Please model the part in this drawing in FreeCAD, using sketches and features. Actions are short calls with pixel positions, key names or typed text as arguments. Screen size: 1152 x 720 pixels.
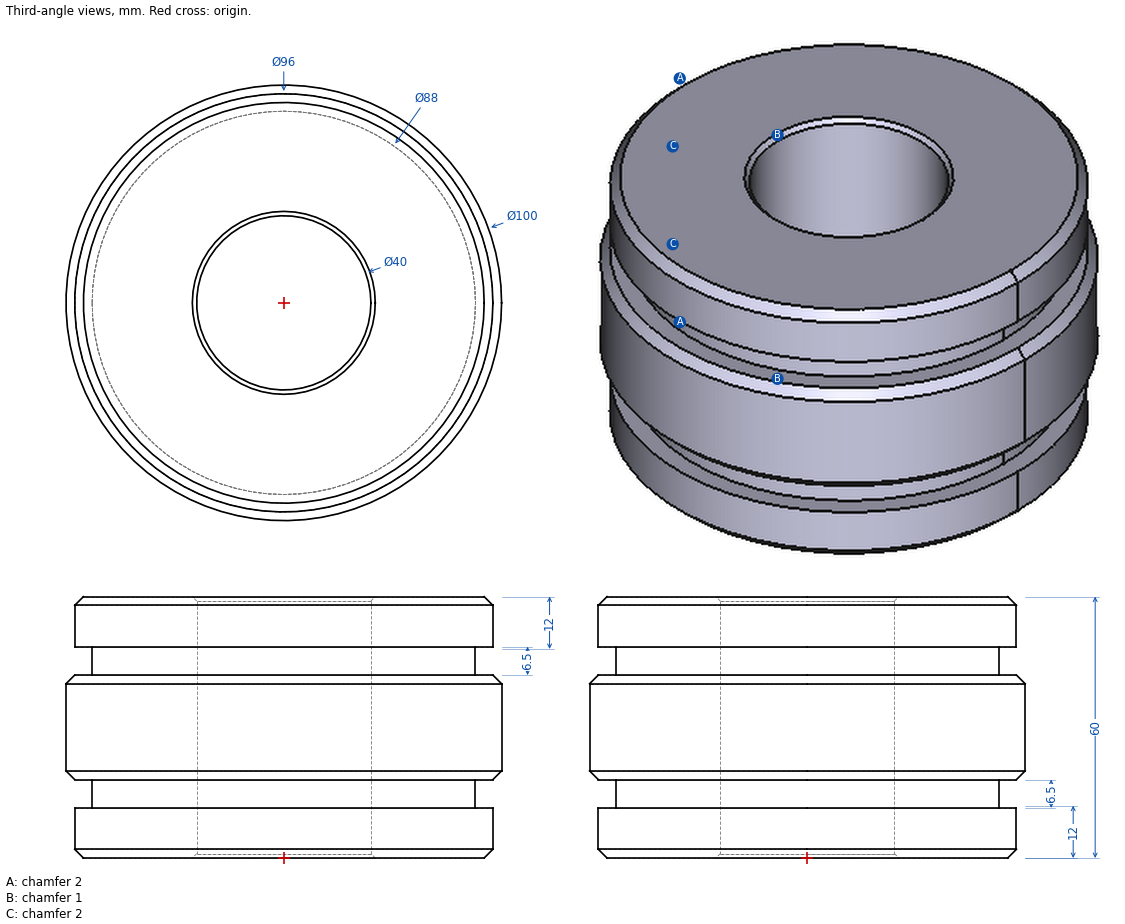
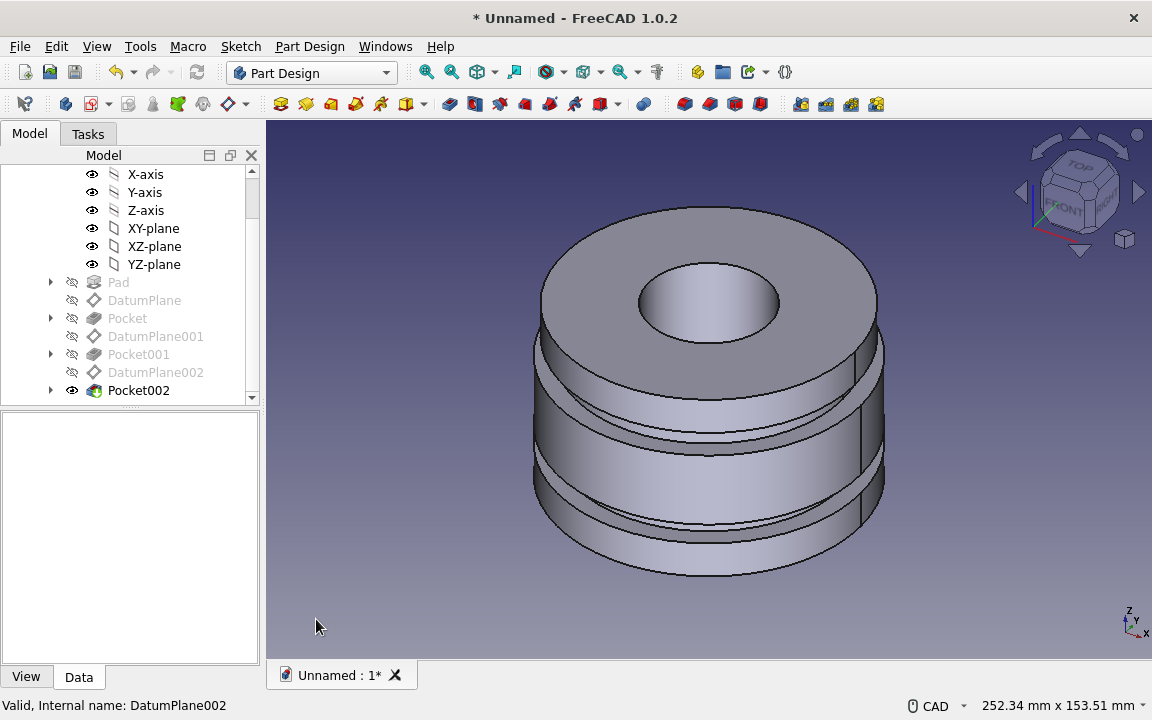
click(90, 104)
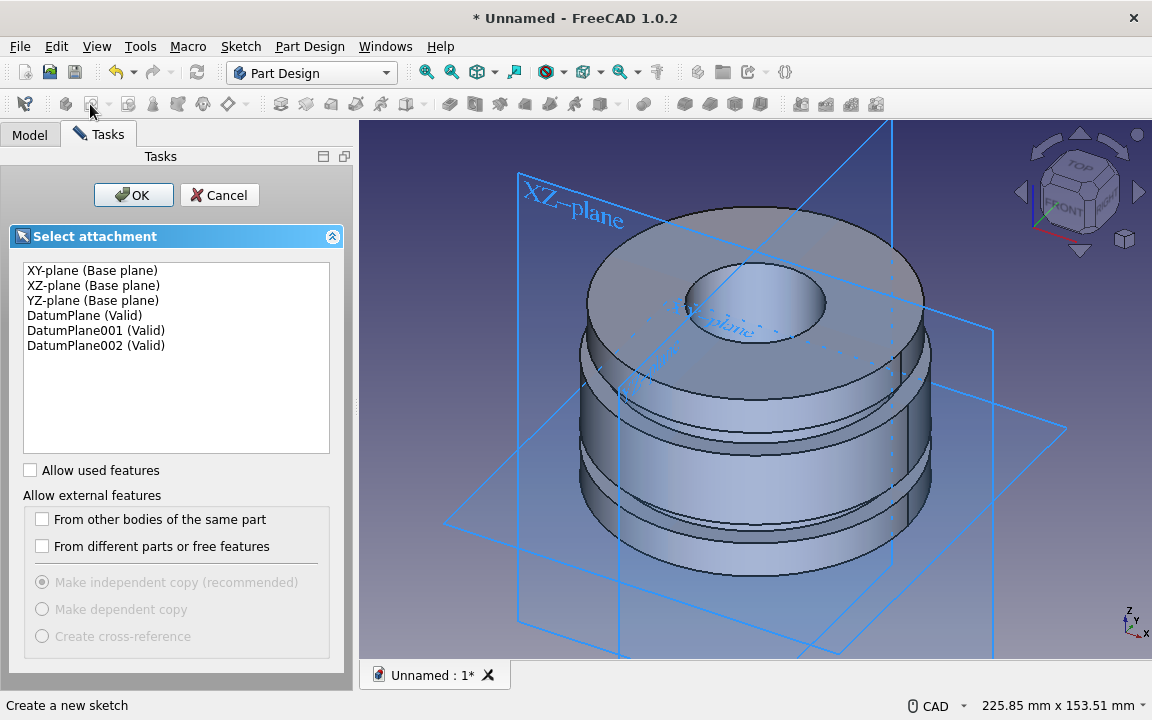
click(84, 270)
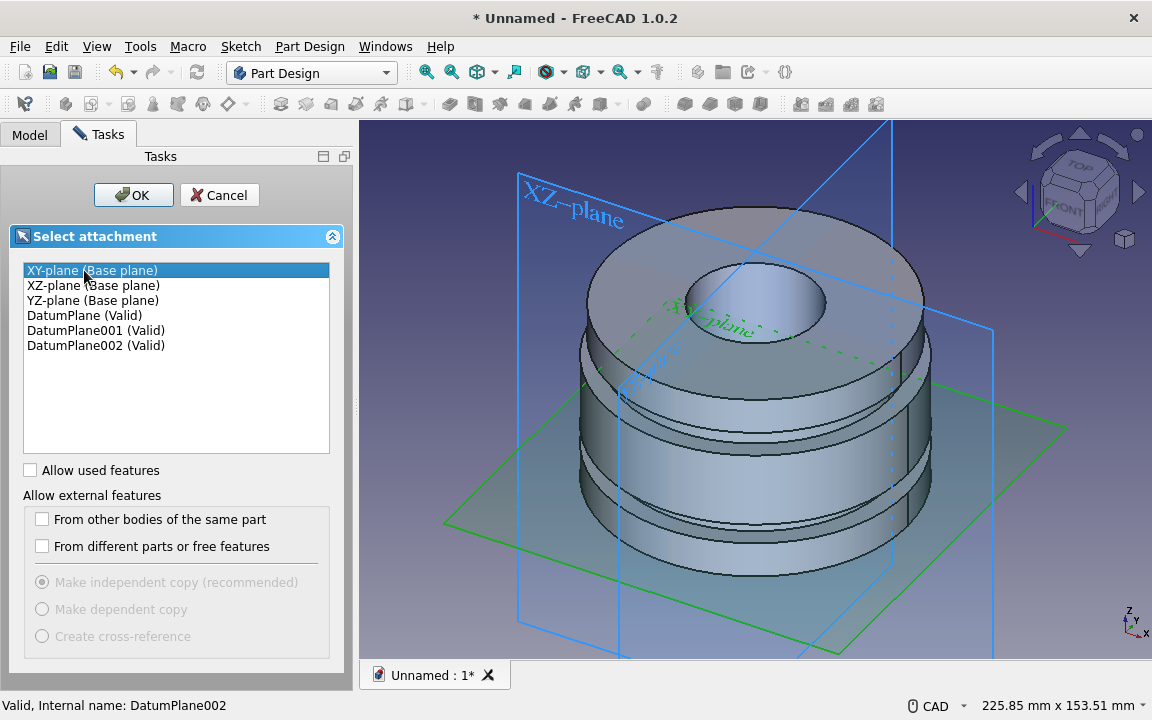
click(134, 195)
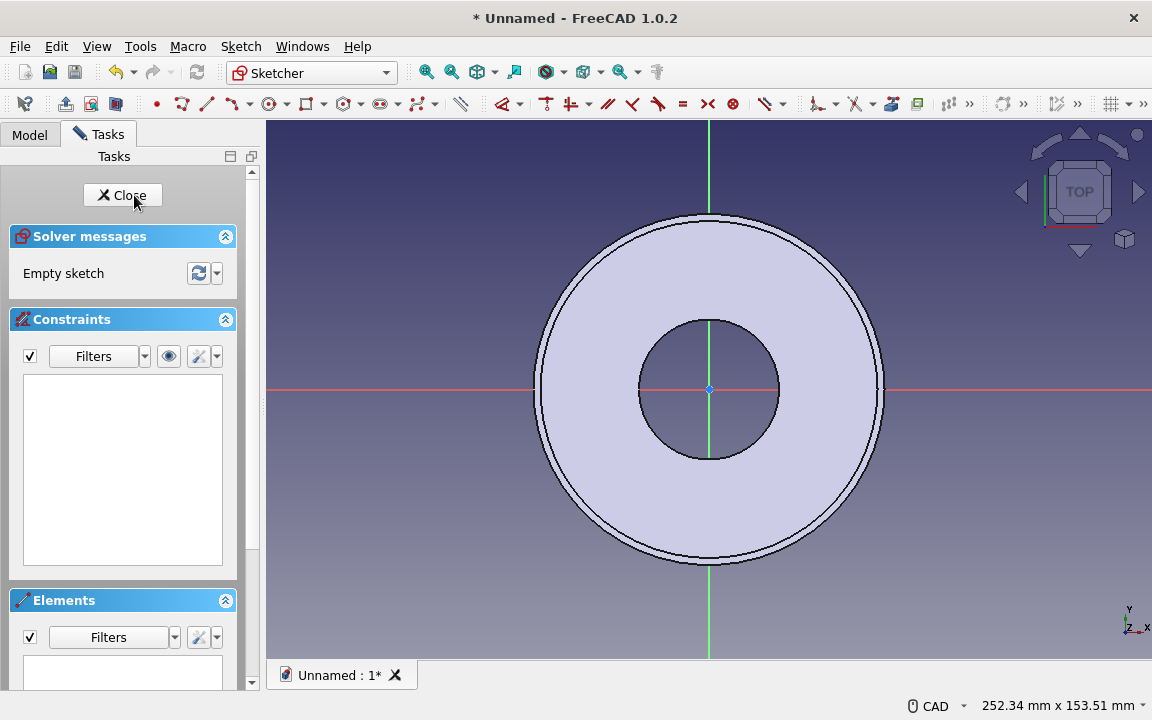
click(116, 104)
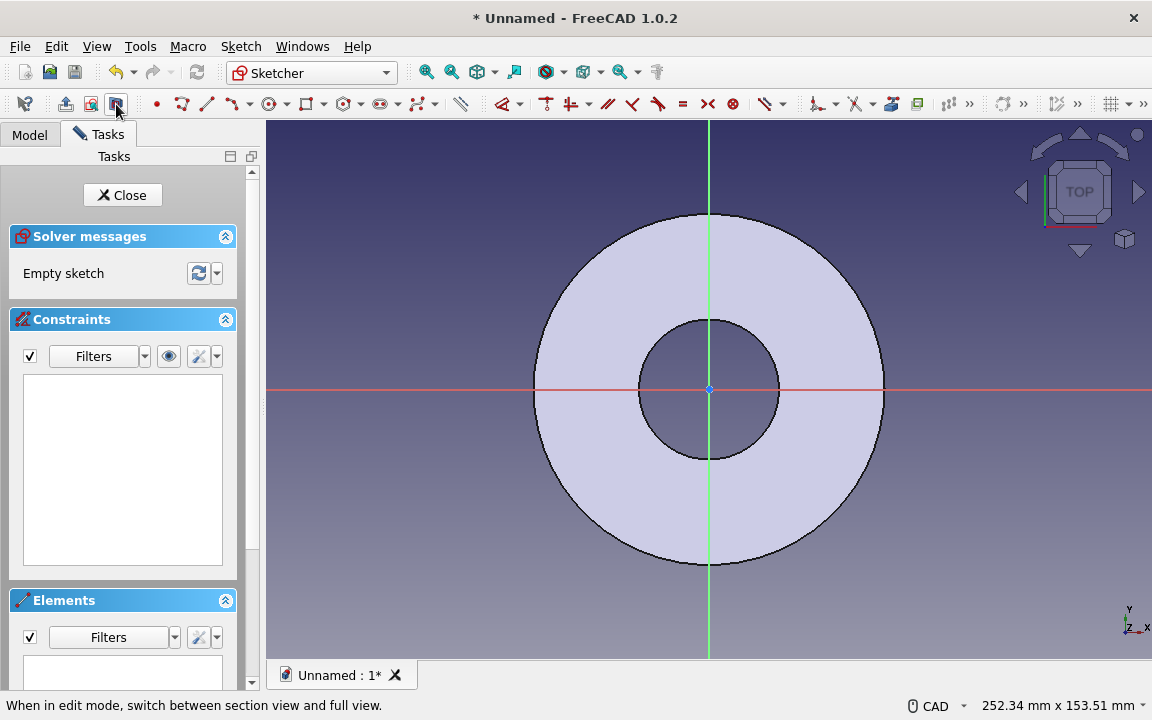
click(268, 104)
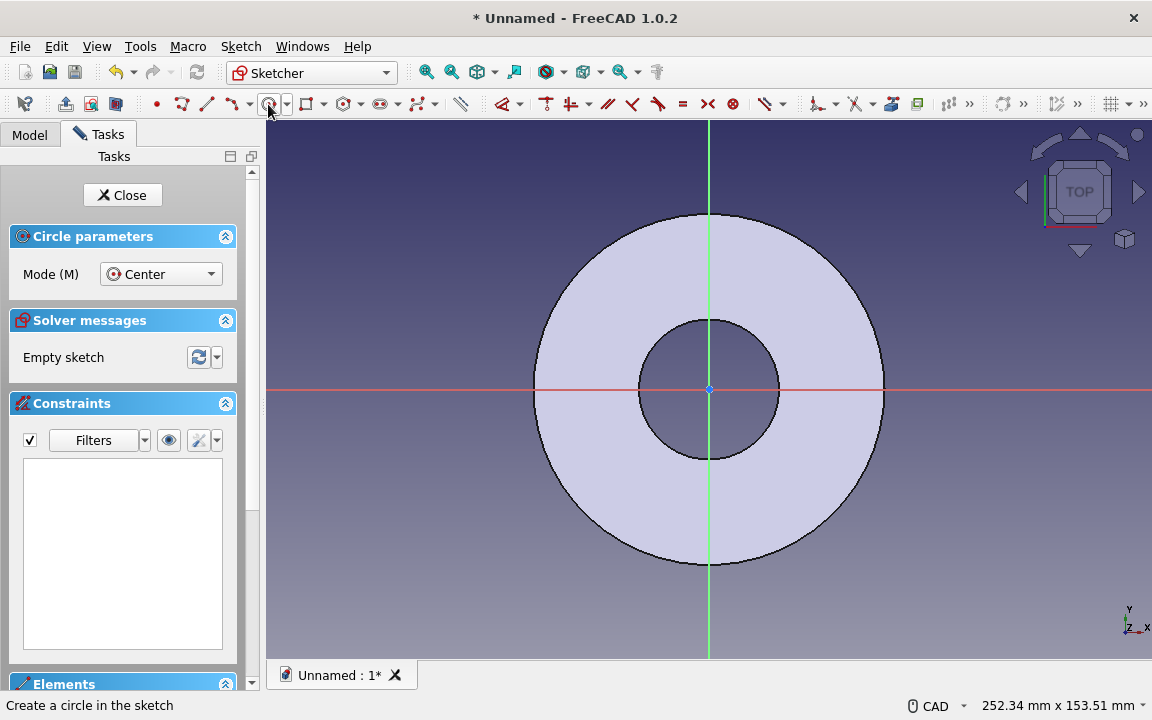
click(709, 390)
click(833, 265)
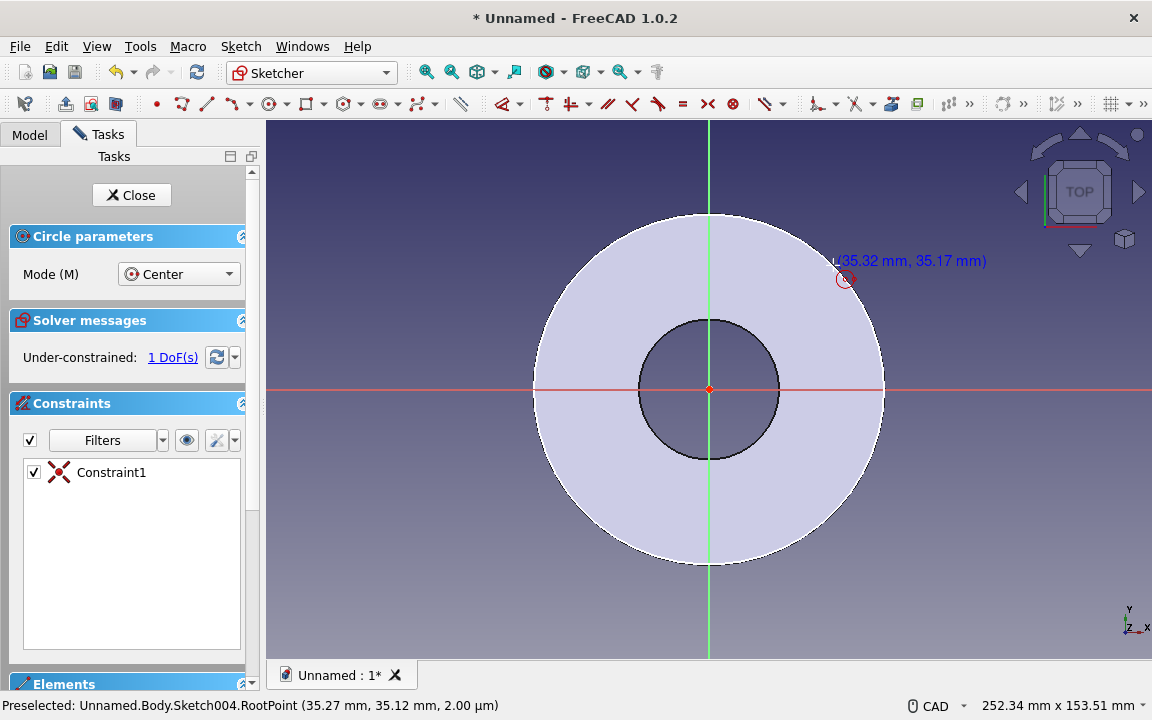
click(709, 390)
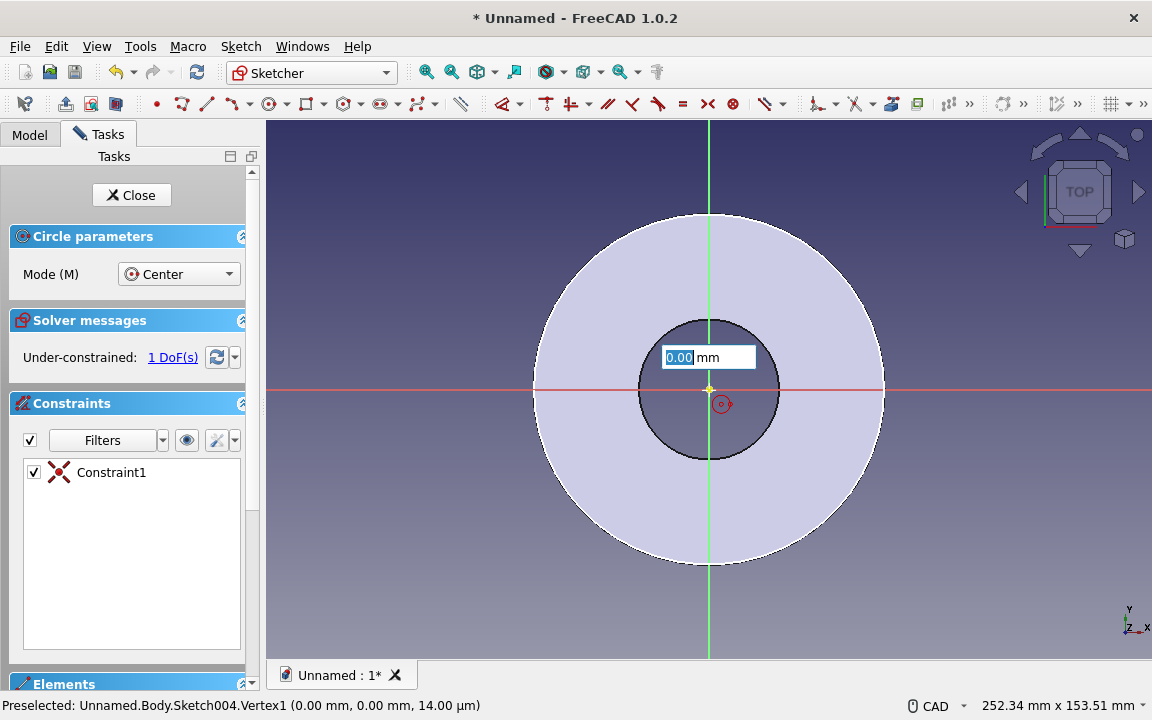
scroll(828, 509, up, 5)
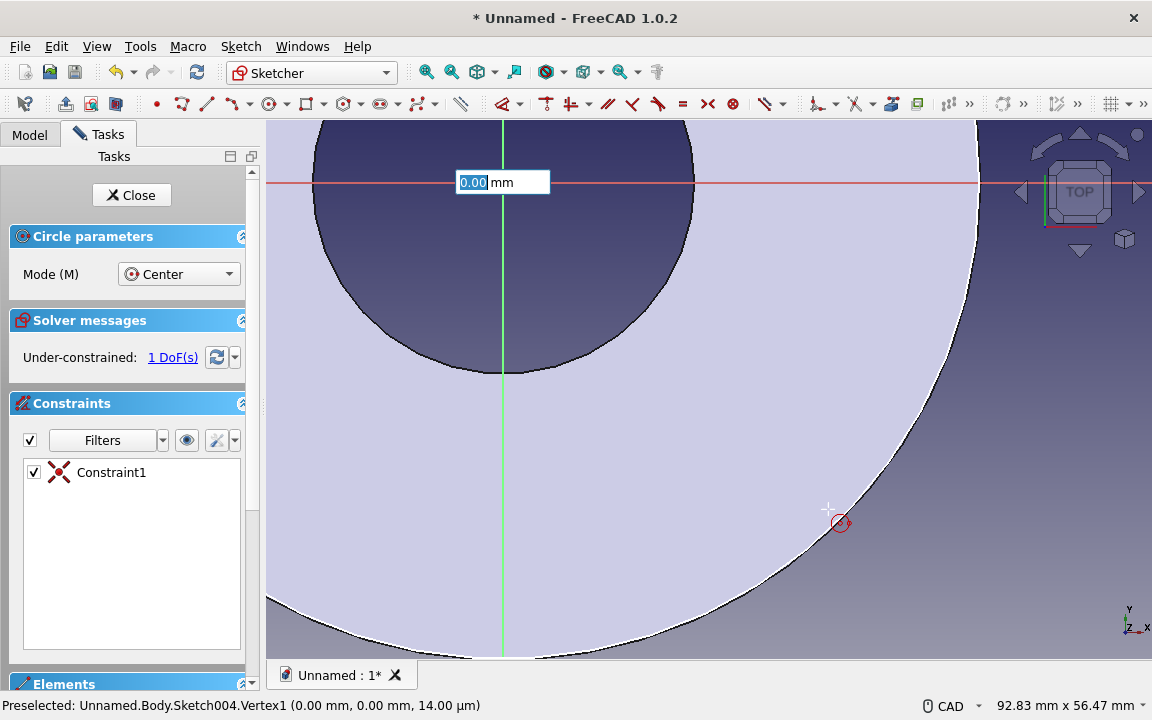
click(827, 507)
key(Escape)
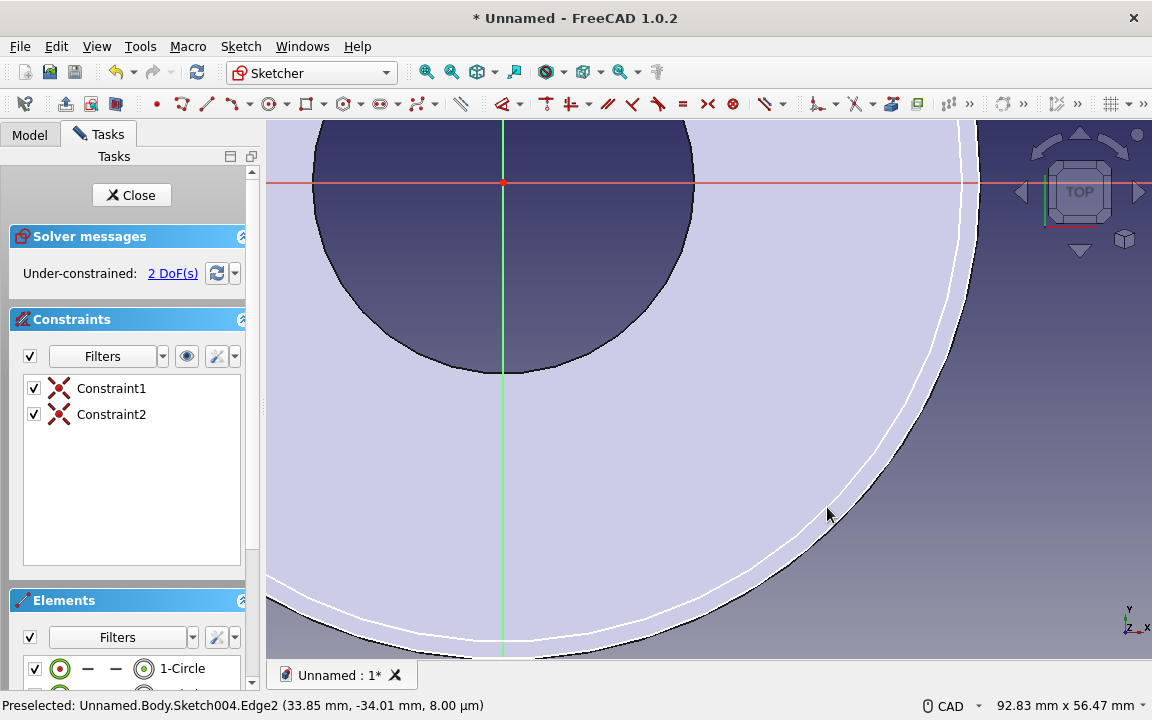
click(502, 104)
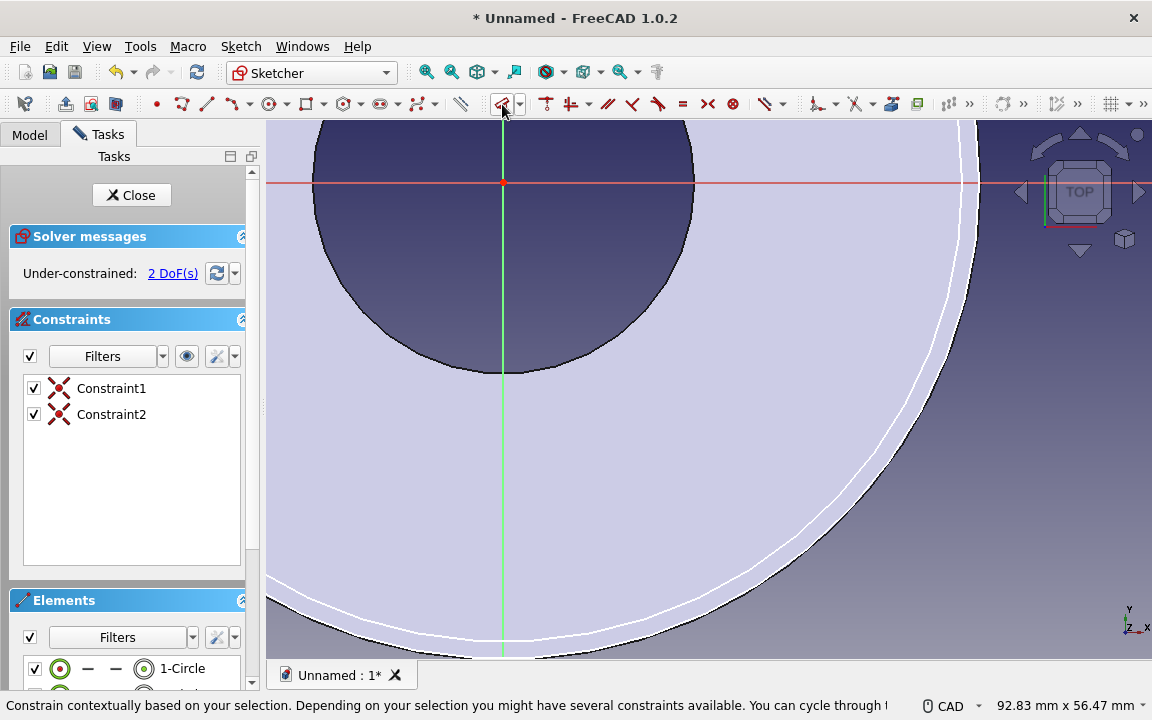
click(841, 518)
click(864, 541)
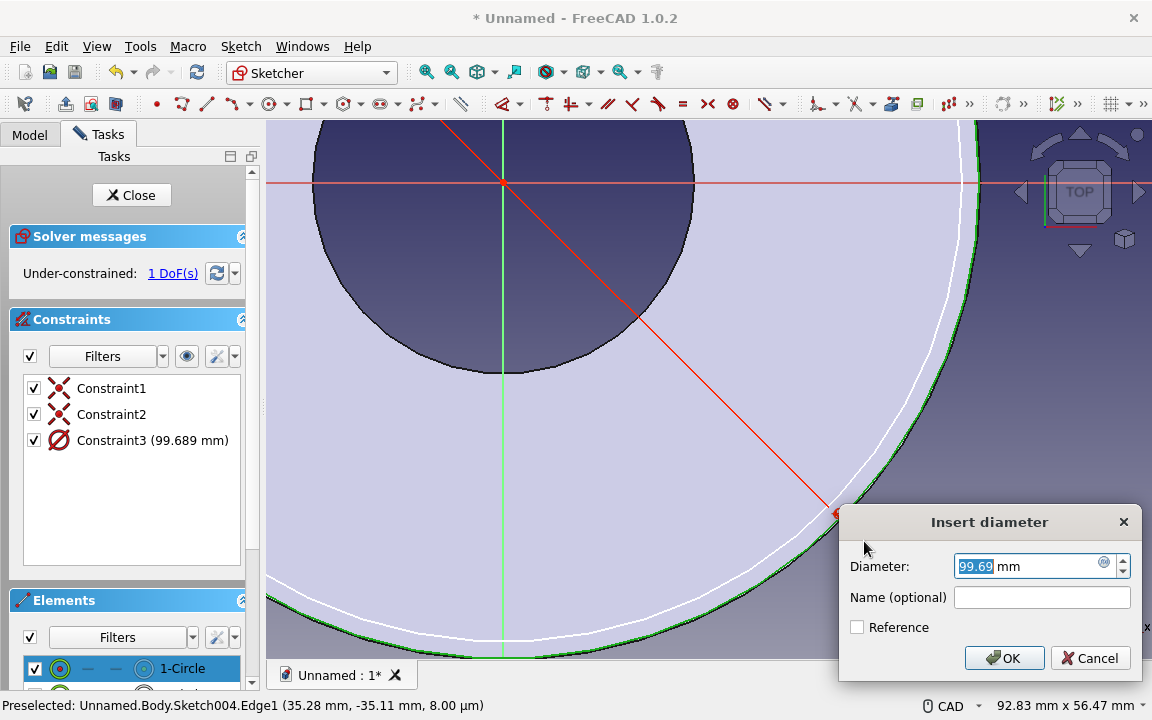
text(100)
key(Return)